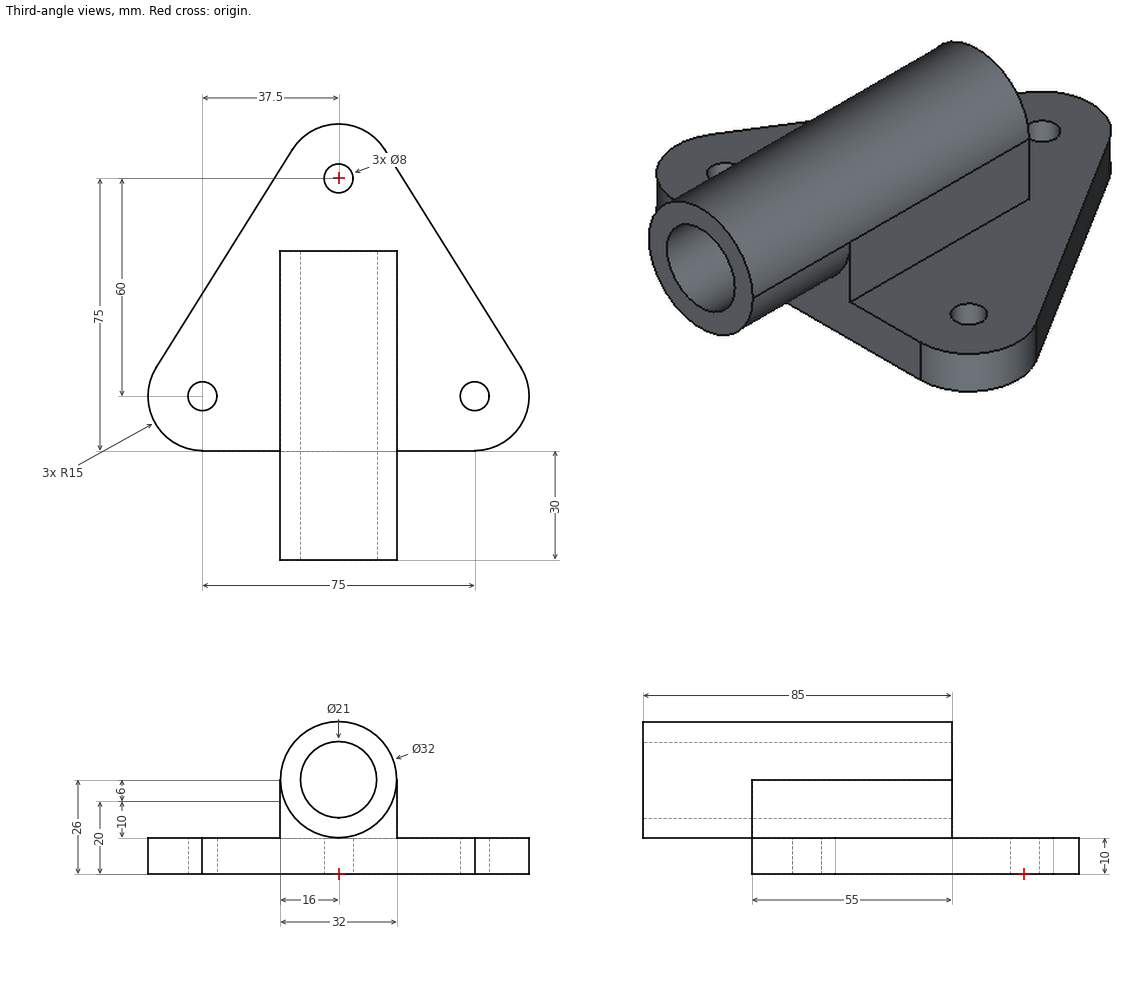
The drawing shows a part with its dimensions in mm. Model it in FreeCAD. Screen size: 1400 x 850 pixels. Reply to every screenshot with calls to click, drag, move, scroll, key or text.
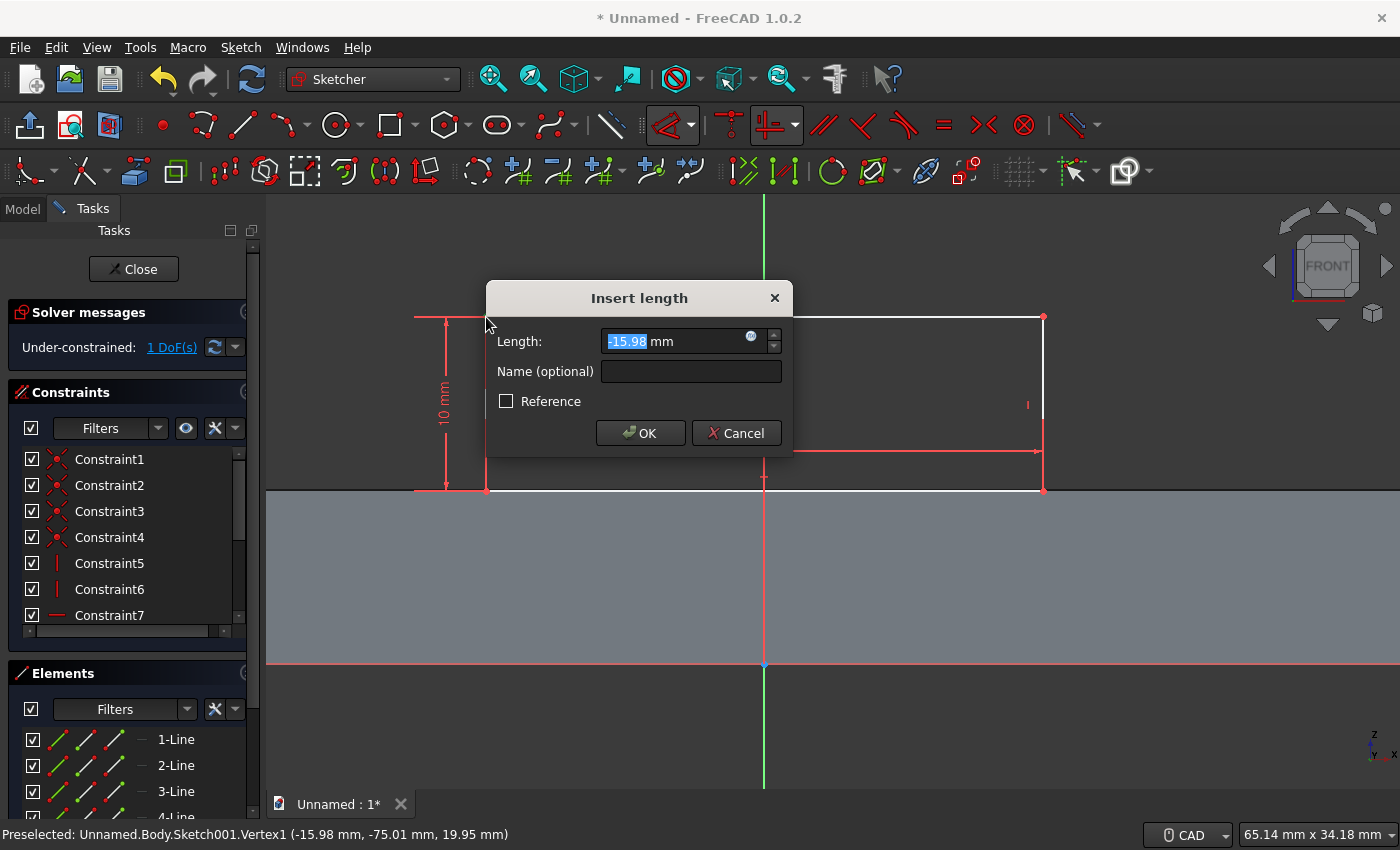
text(-16)
key(Return)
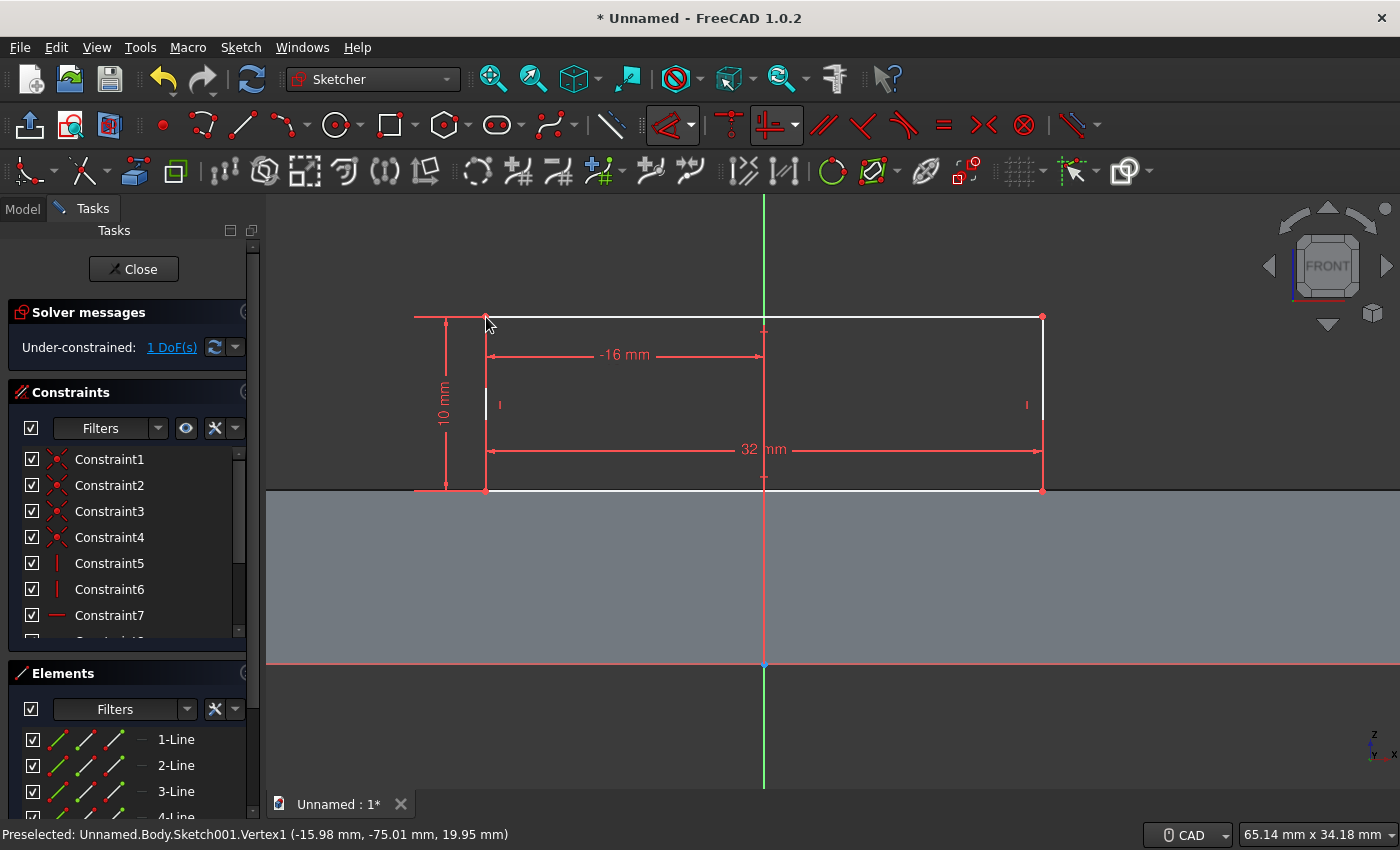
click(486, 317)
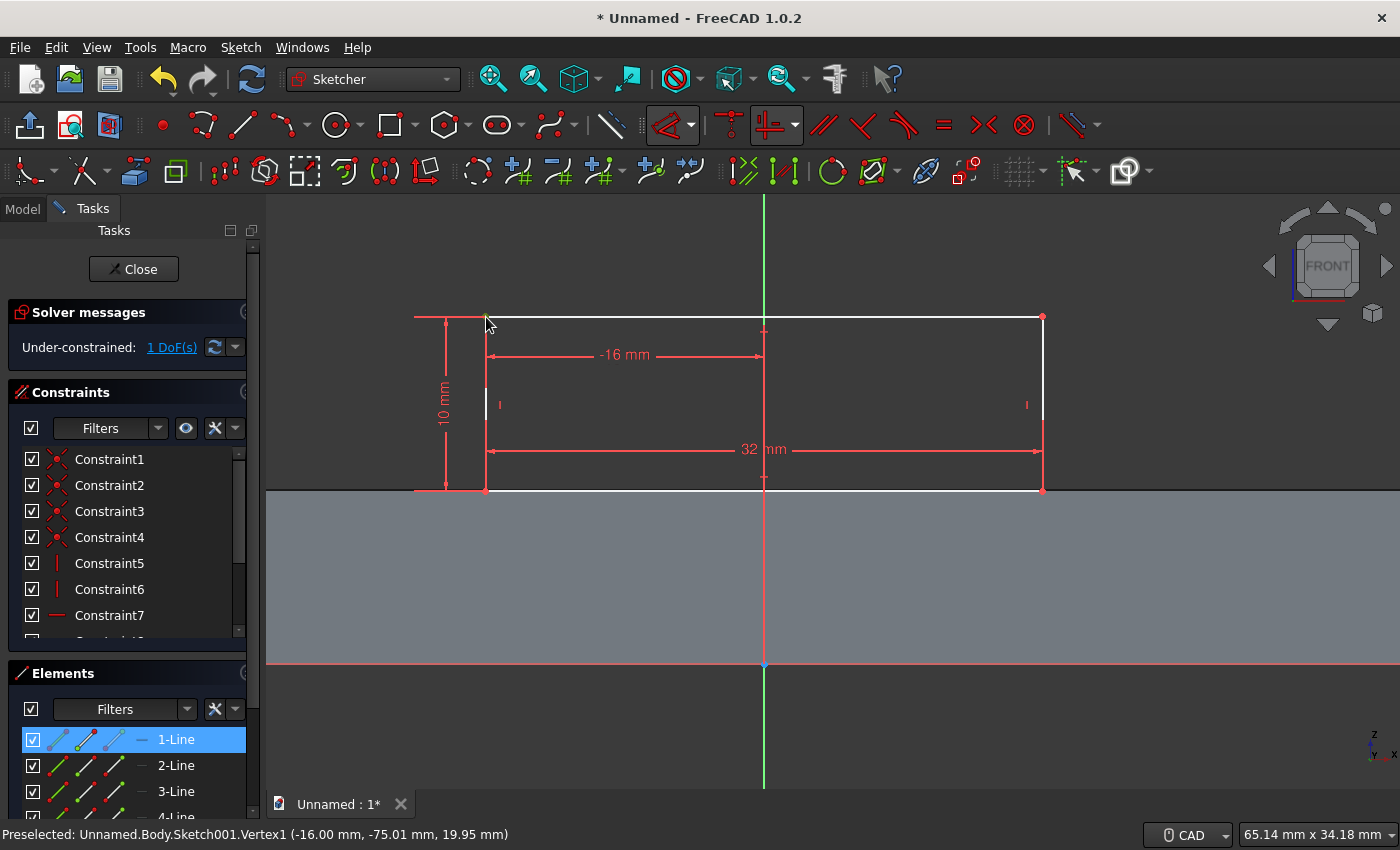
key(i)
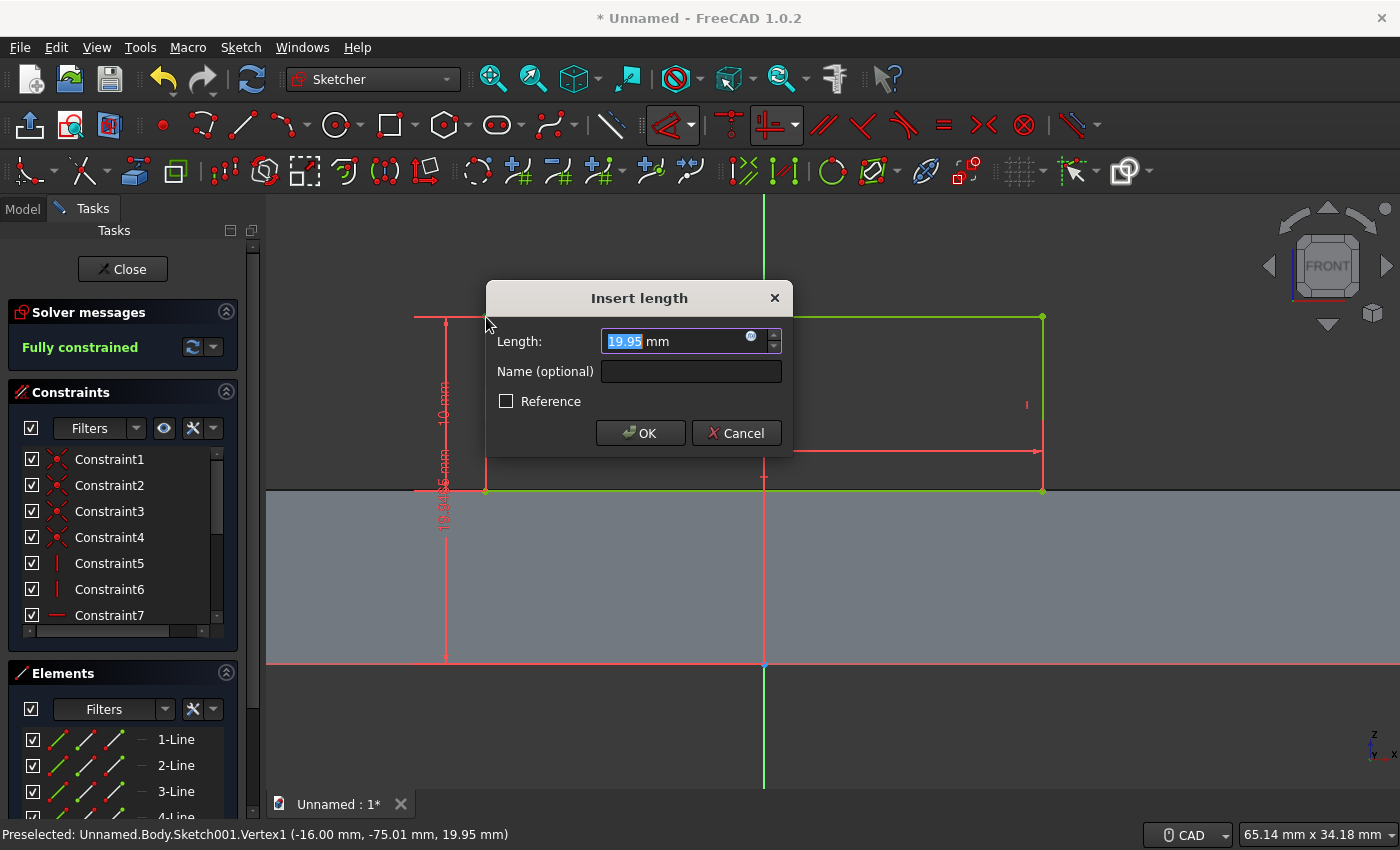
text(20)
key(Return)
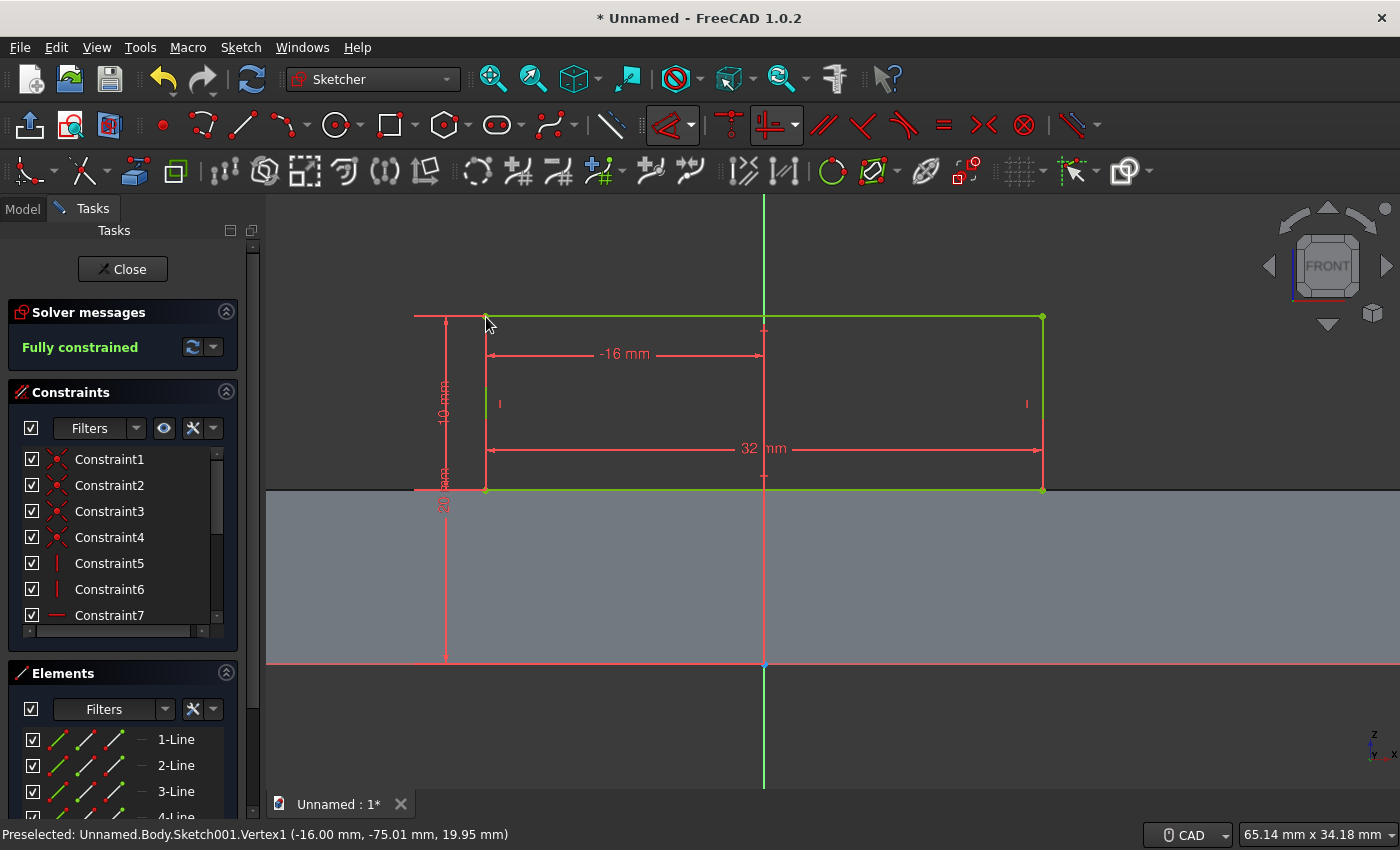
click(123, 269)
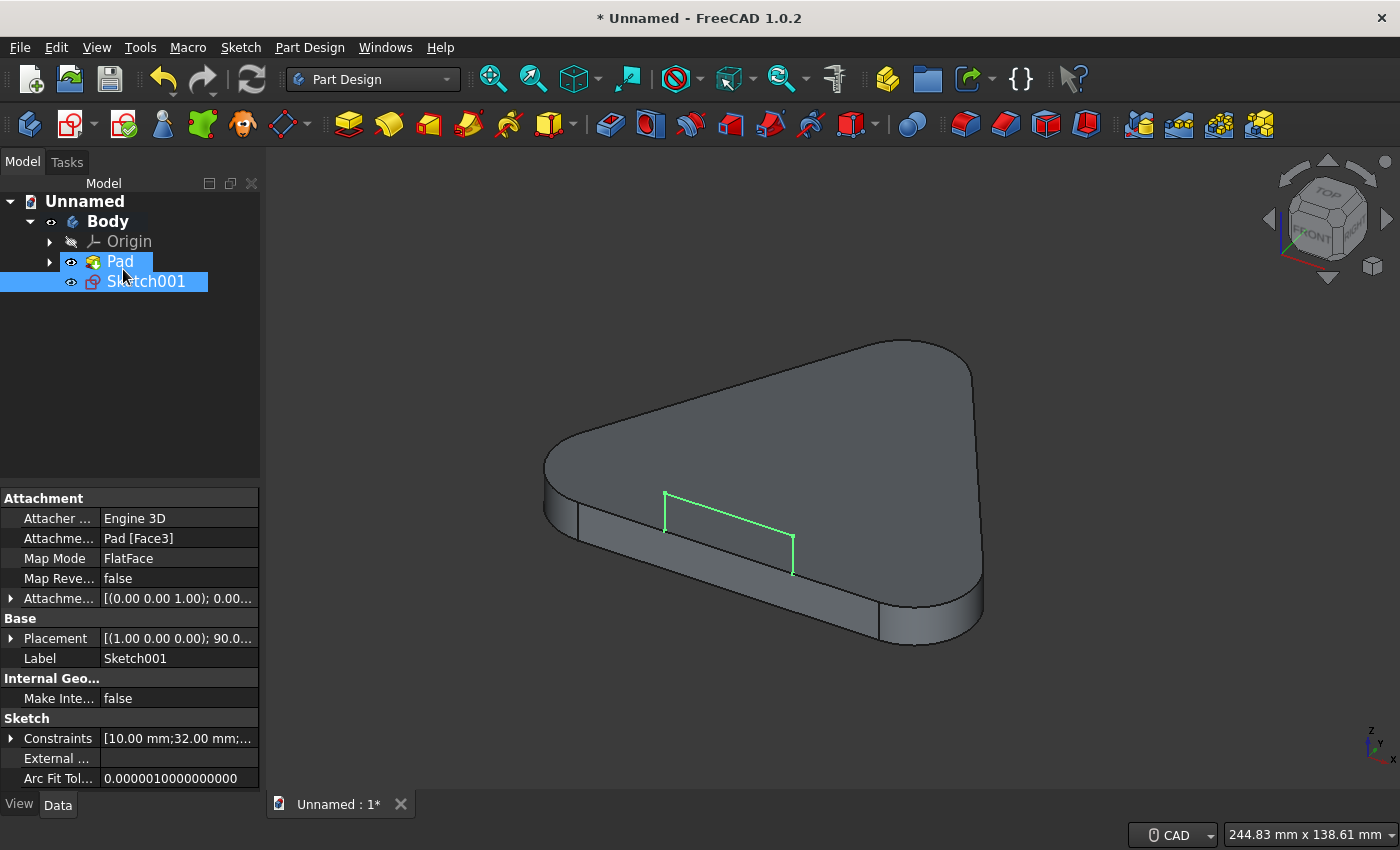
click(350, 124)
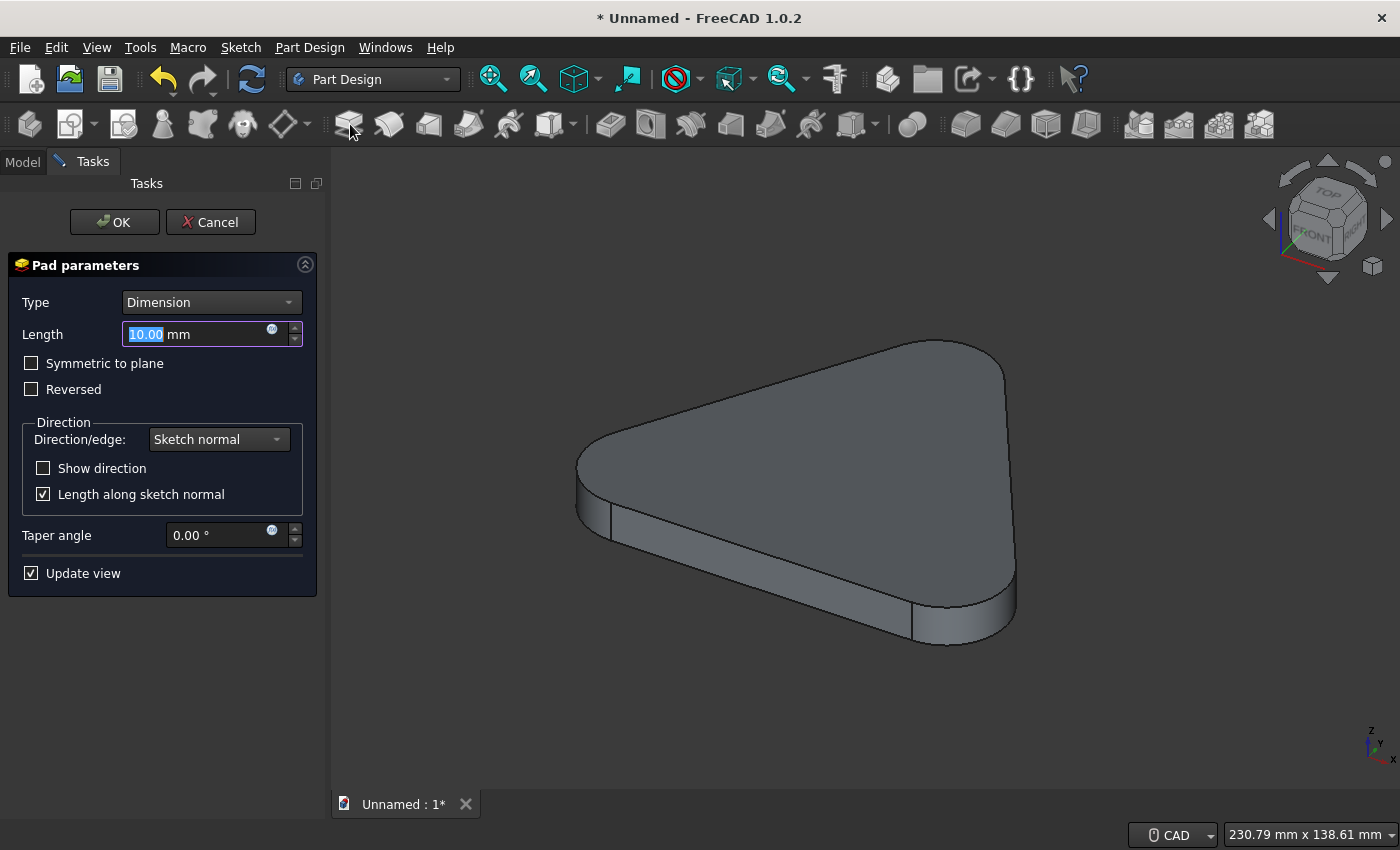
text(55)
key(Tab)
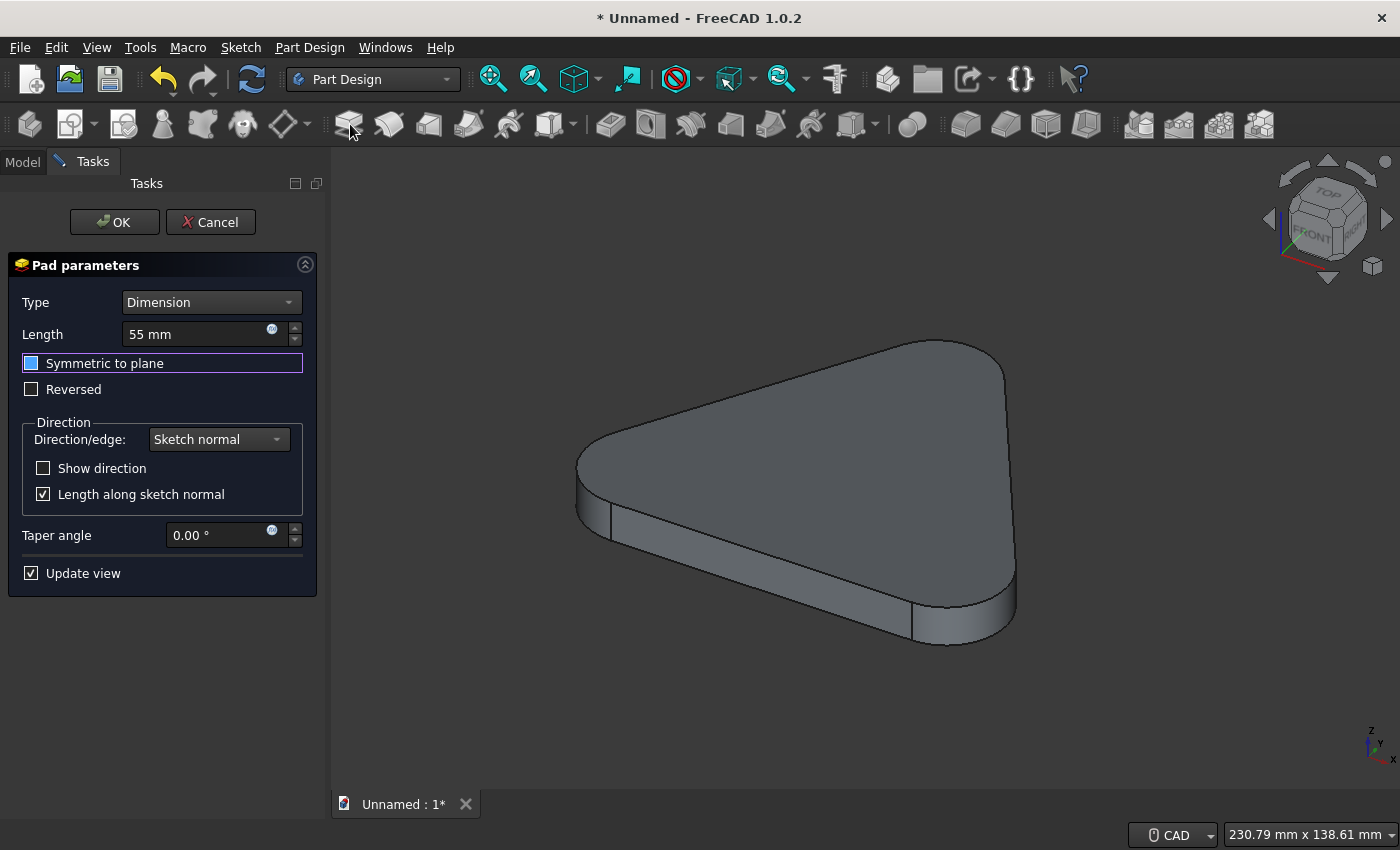
click(30, 389)